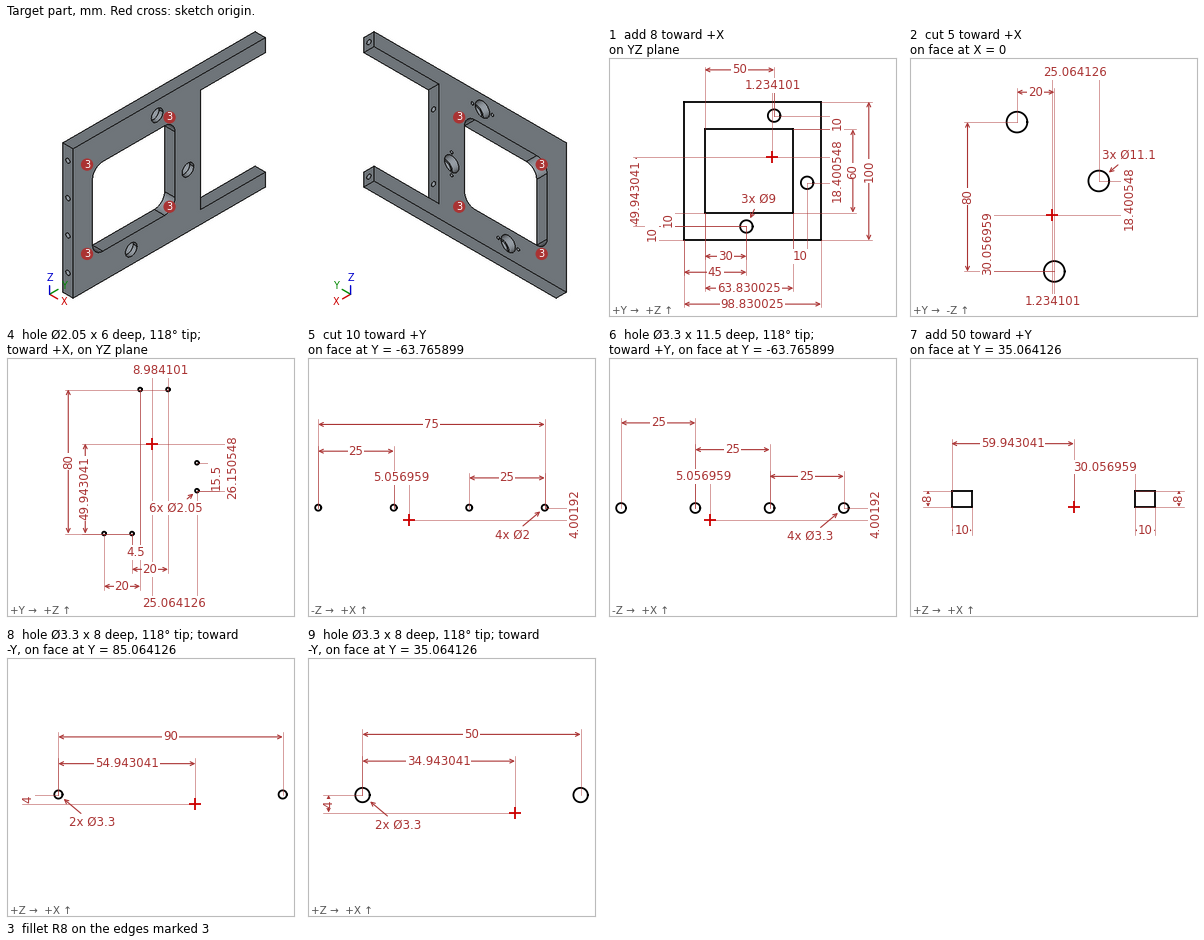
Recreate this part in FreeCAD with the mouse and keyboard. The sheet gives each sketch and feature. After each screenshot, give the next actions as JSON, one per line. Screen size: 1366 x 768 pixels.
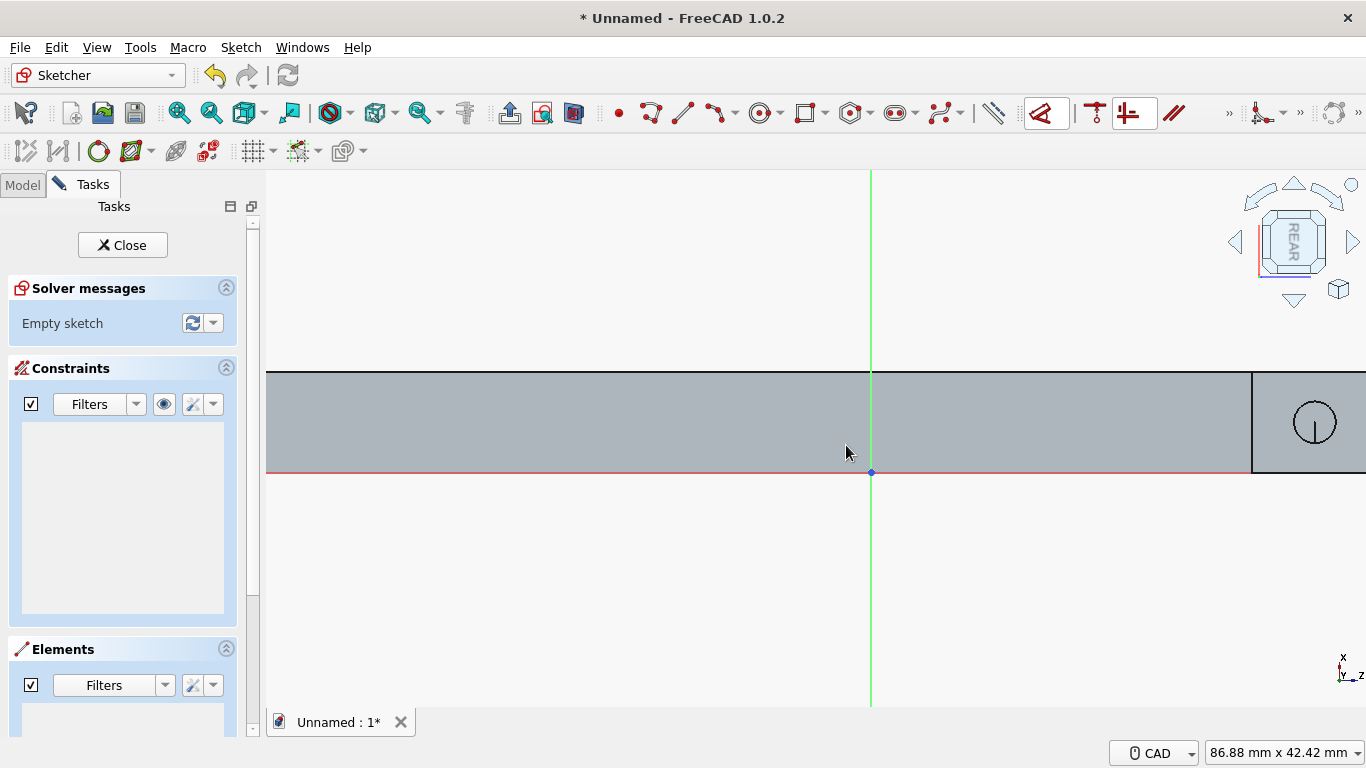
{"action": "key", "text": "g c"}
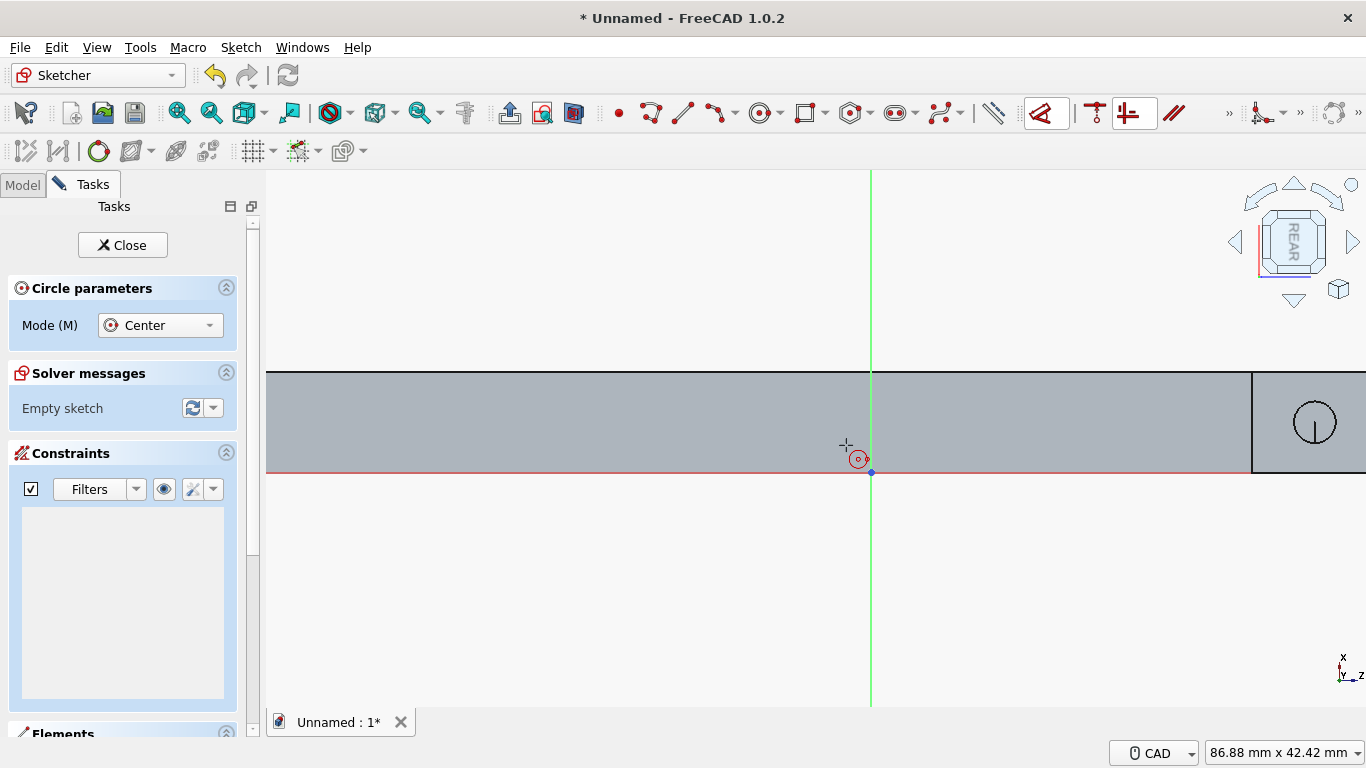
{"action": "left_click", "coordinate": [429, 422]}
{"action": "mouse_move", "coordinate": [443, 407]}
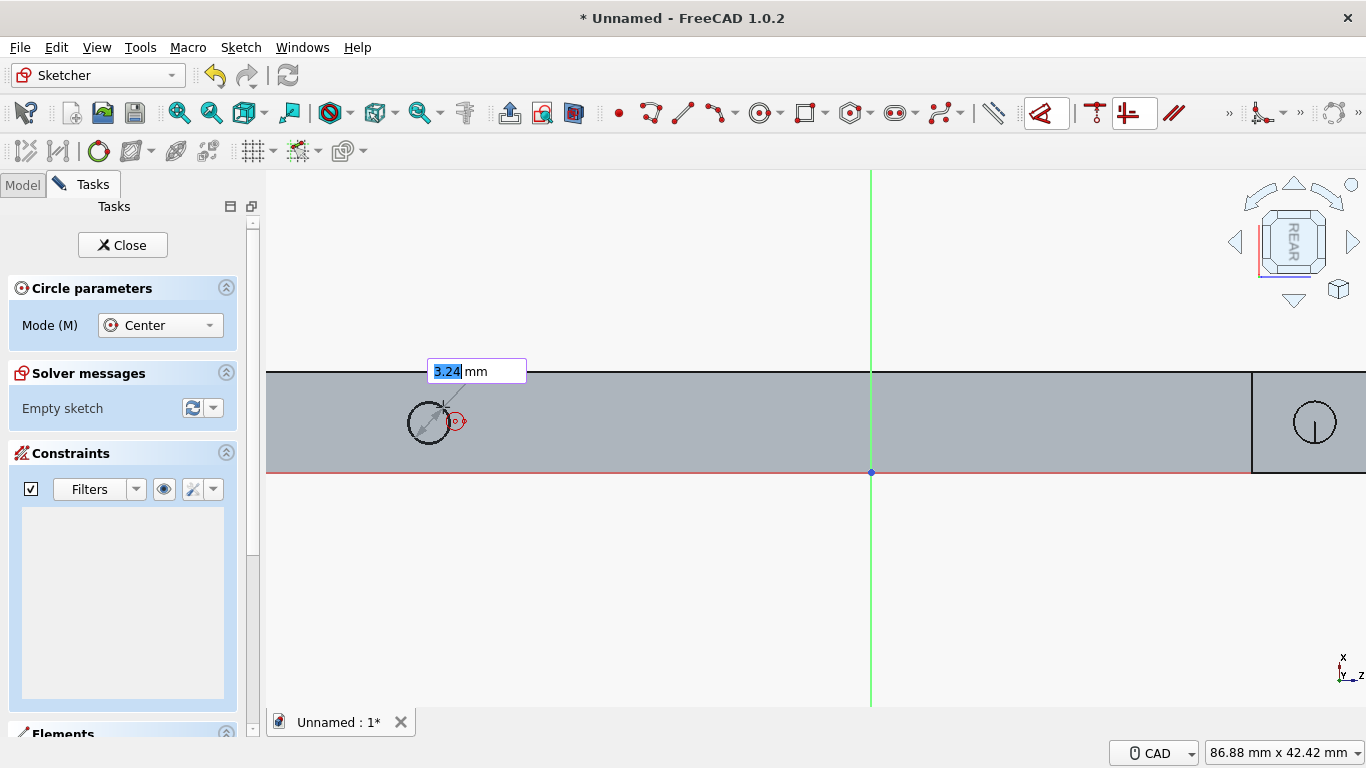
{"action": "type", "text": "3.3"}
{"action": "key", "text": "Return"}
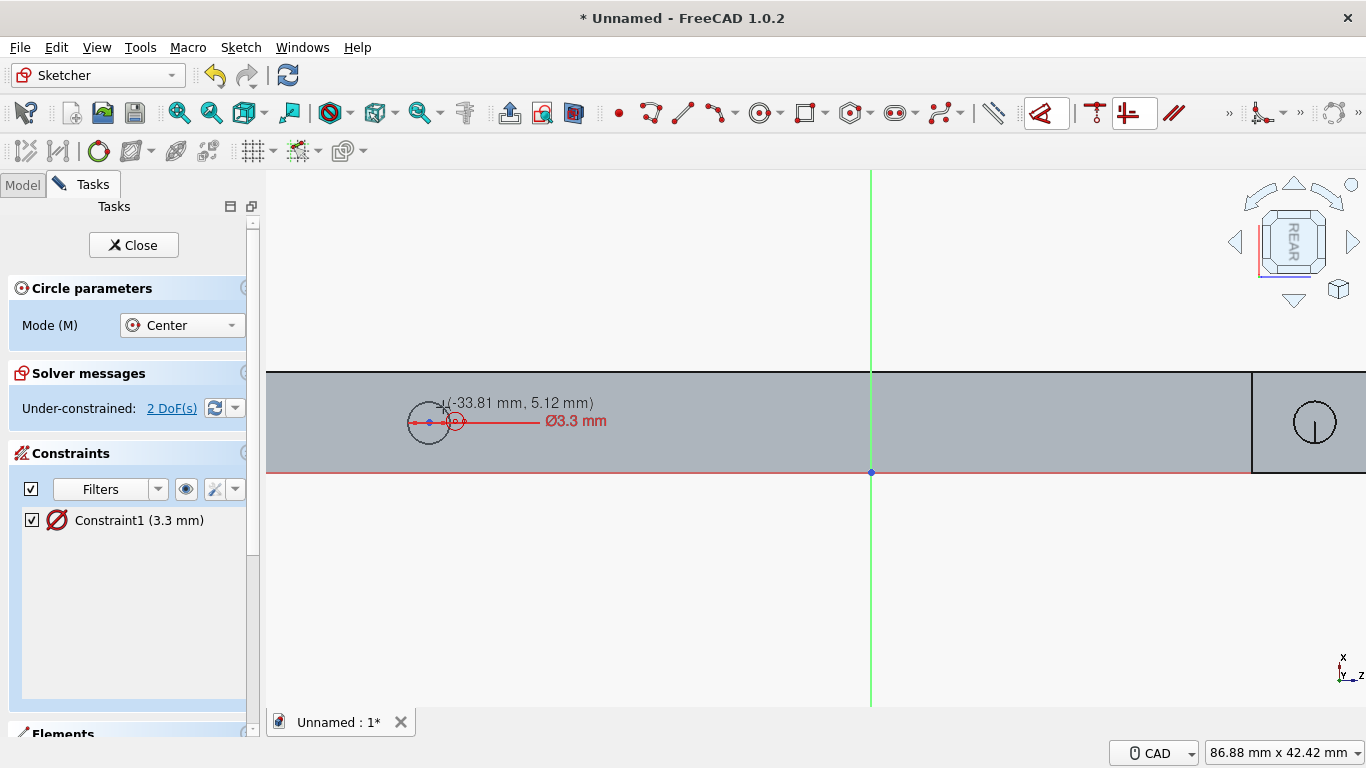
{"action": "left_click", "coordinate": [1062, 422]}
{"action": "mouse_move", "coordinate": [1076, 407]}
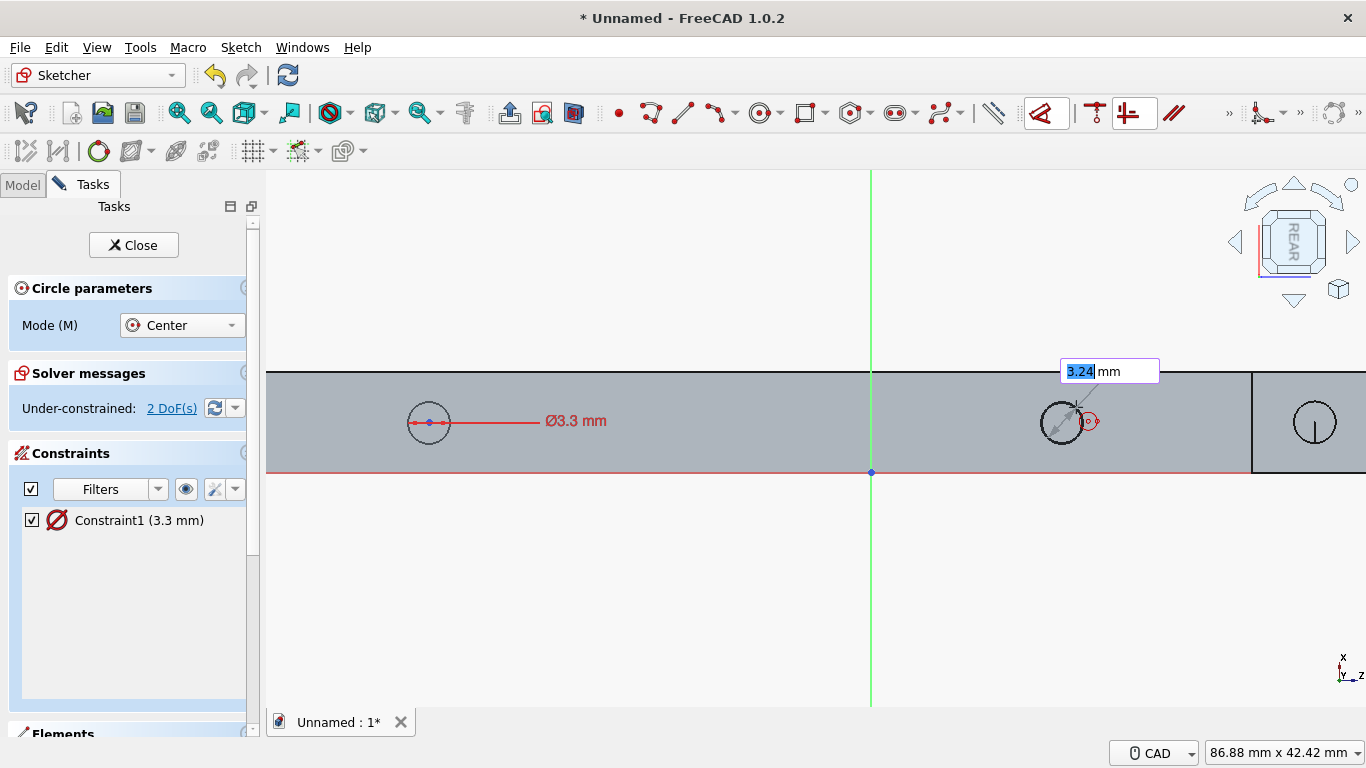
{"action": "type", "text": "3.3"}
{"action": "key", "text": "Return"}
{"action": "key", "text": "Escape"}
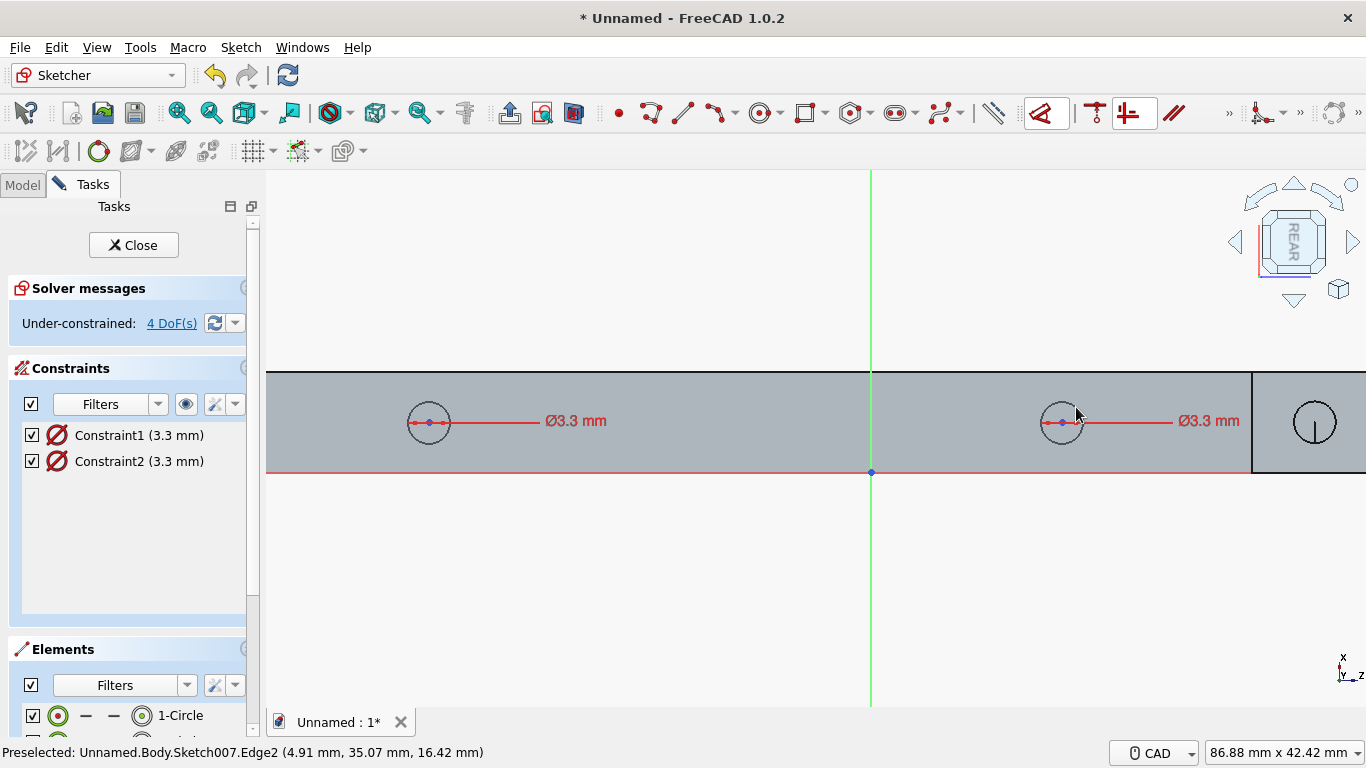
{"action": "left_click", "coordinate": [429, 423]}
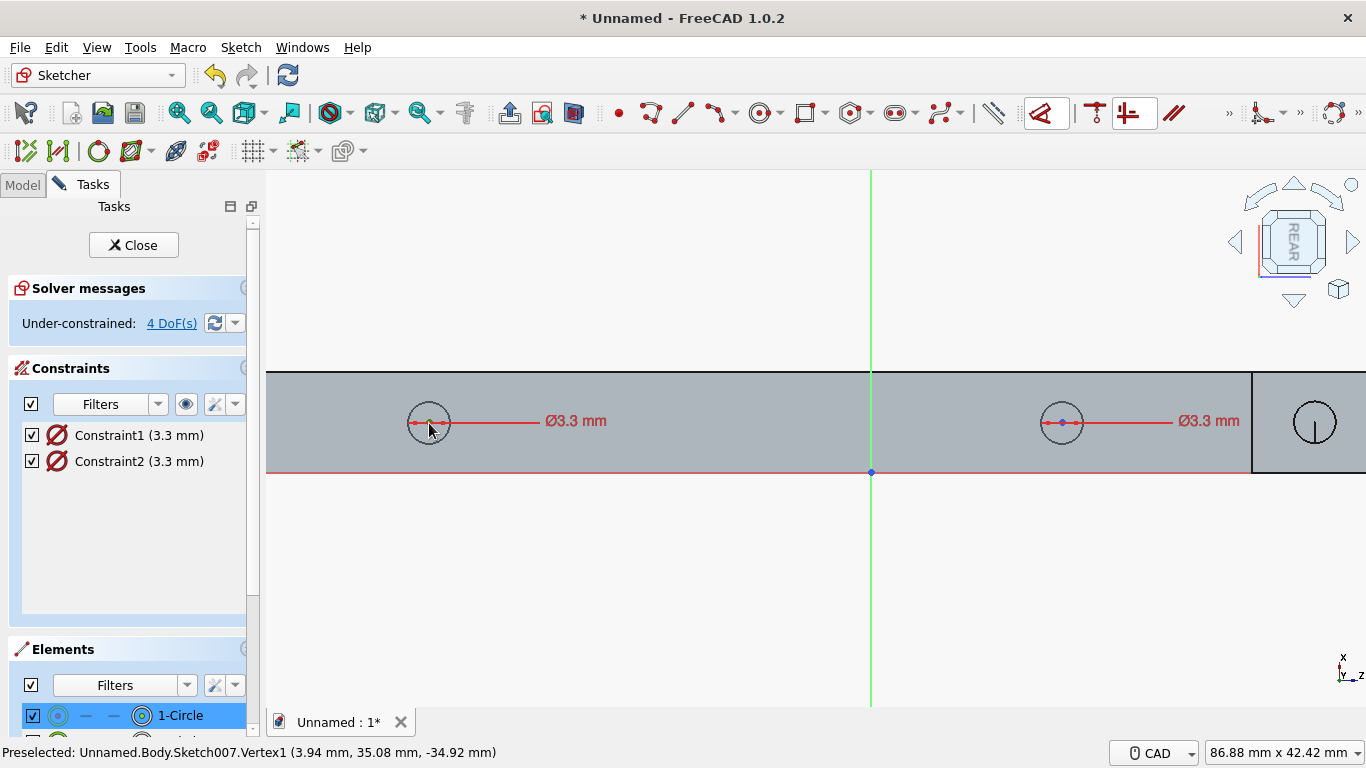
{"action": "left_click", "coordinate": [1062, 423]}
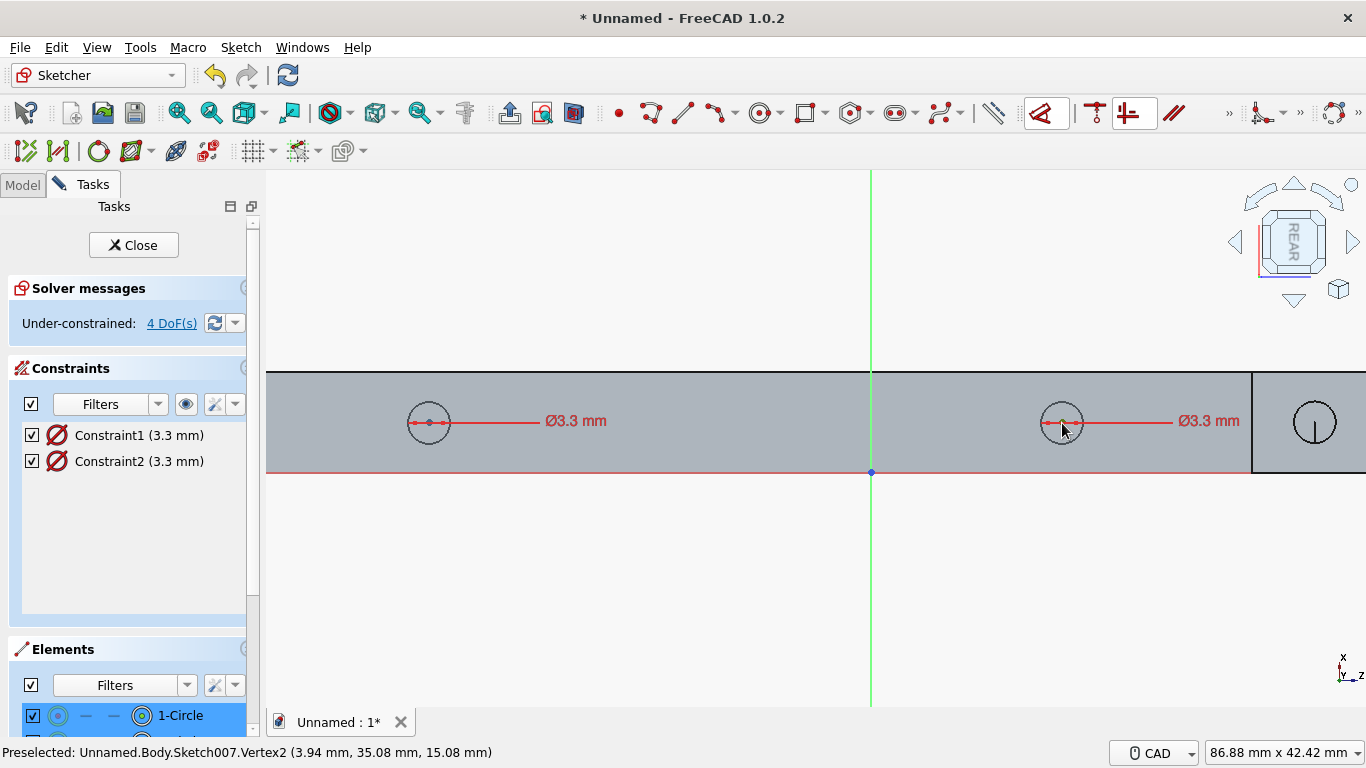
{"action": "left_click", "coordinate": [1152, 114]}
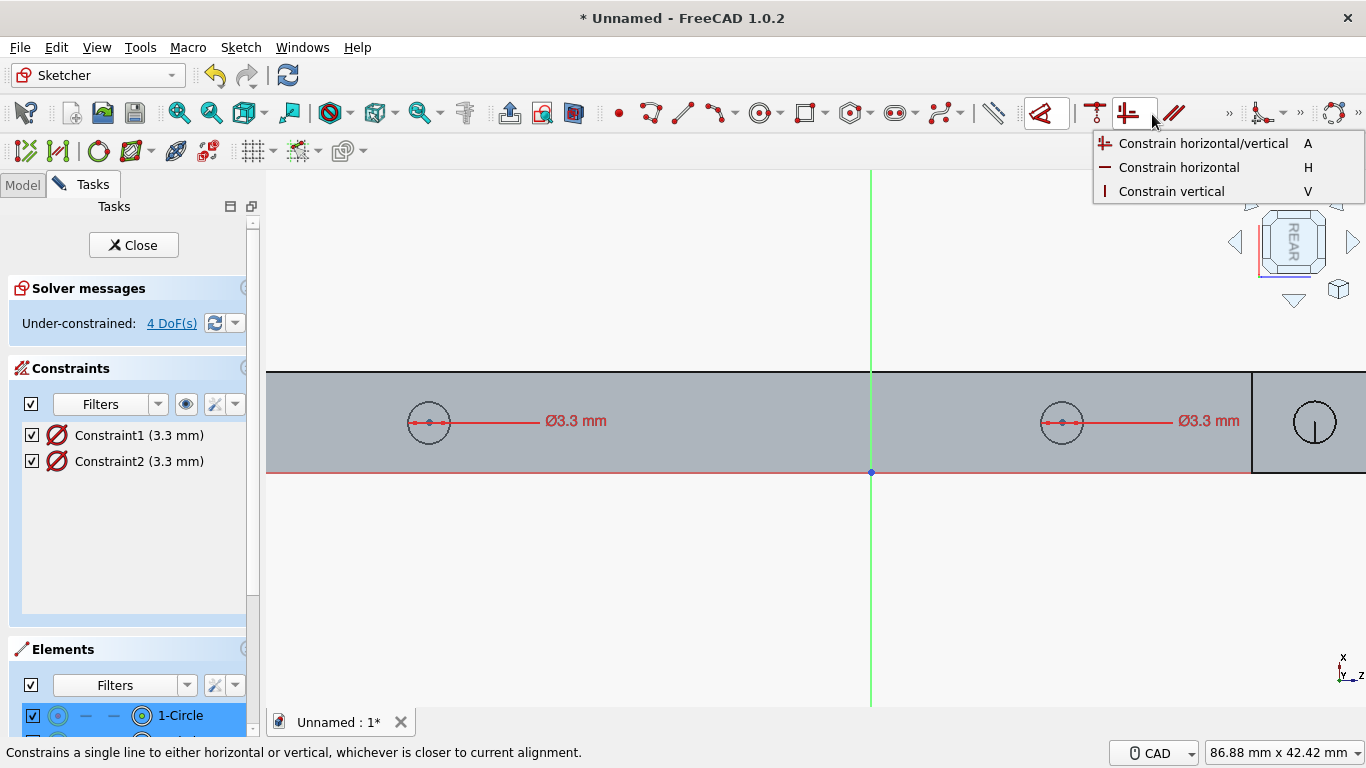
{"action": "left_click", "coordinate": [1229, 167]}